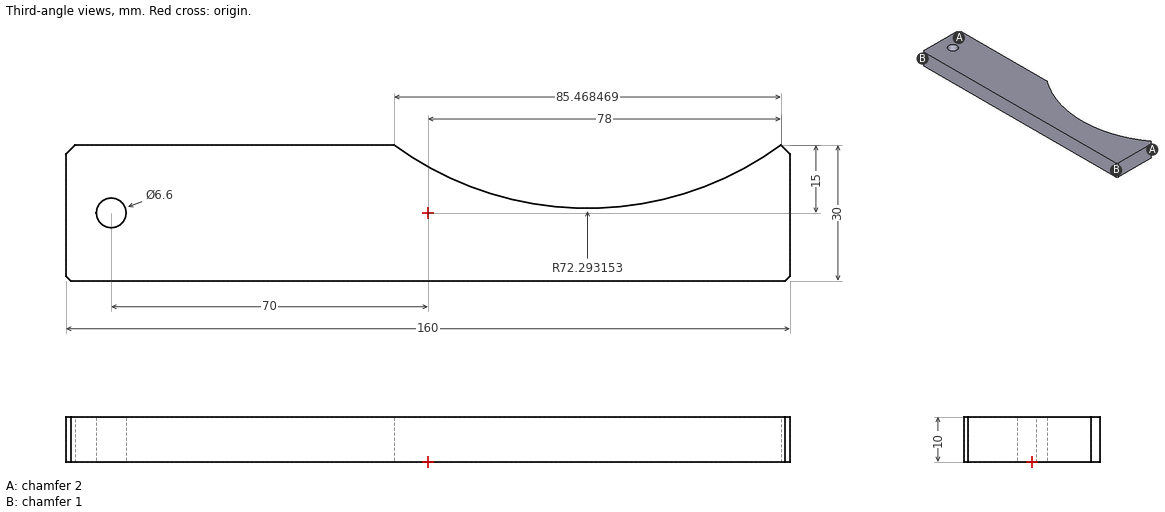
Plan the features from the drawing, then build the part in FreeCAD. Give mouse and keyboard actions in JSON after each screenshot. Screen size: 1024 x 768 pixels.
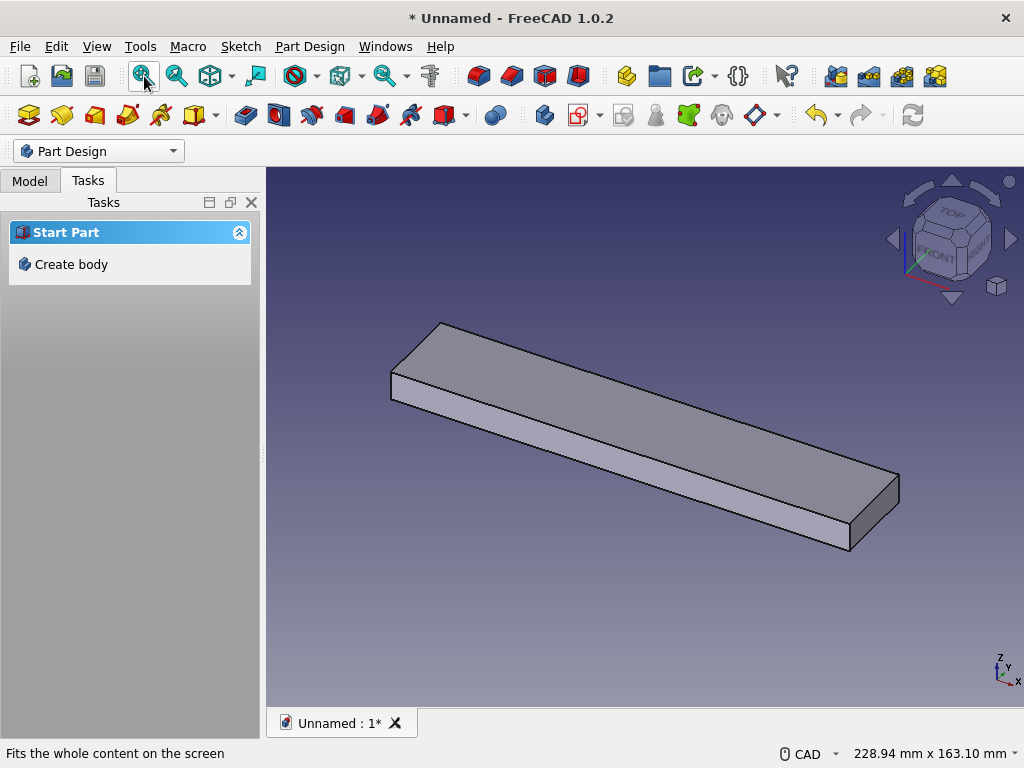
{"action": "key", "text": "0"}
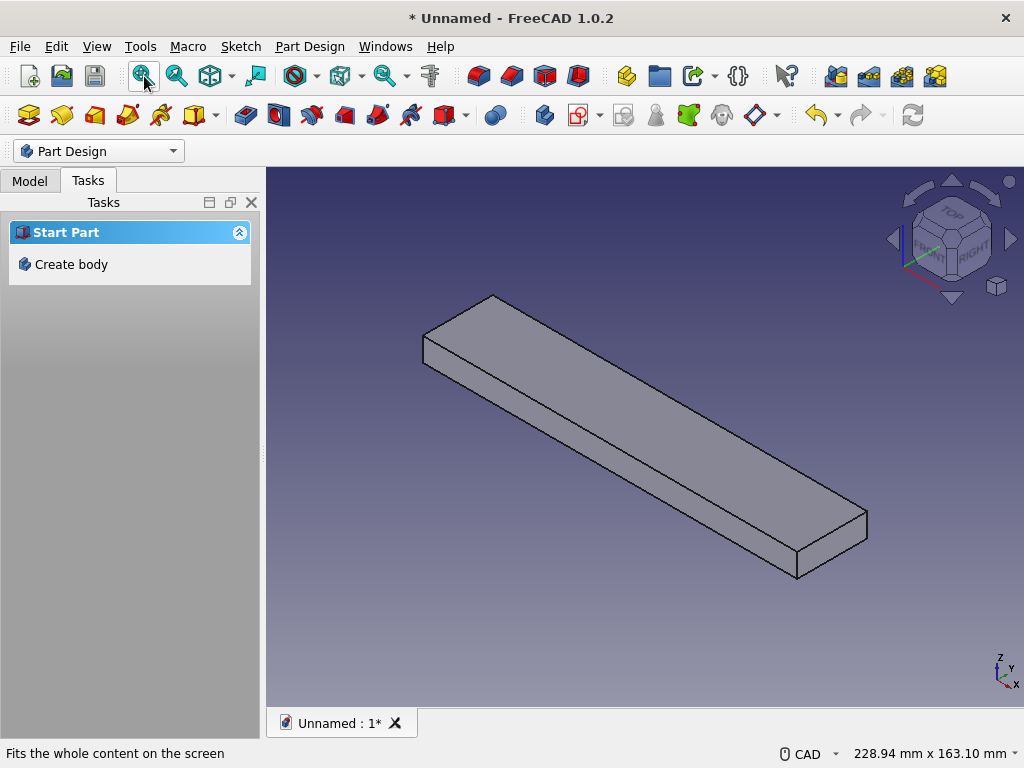
{"action": "key", "text": "2"}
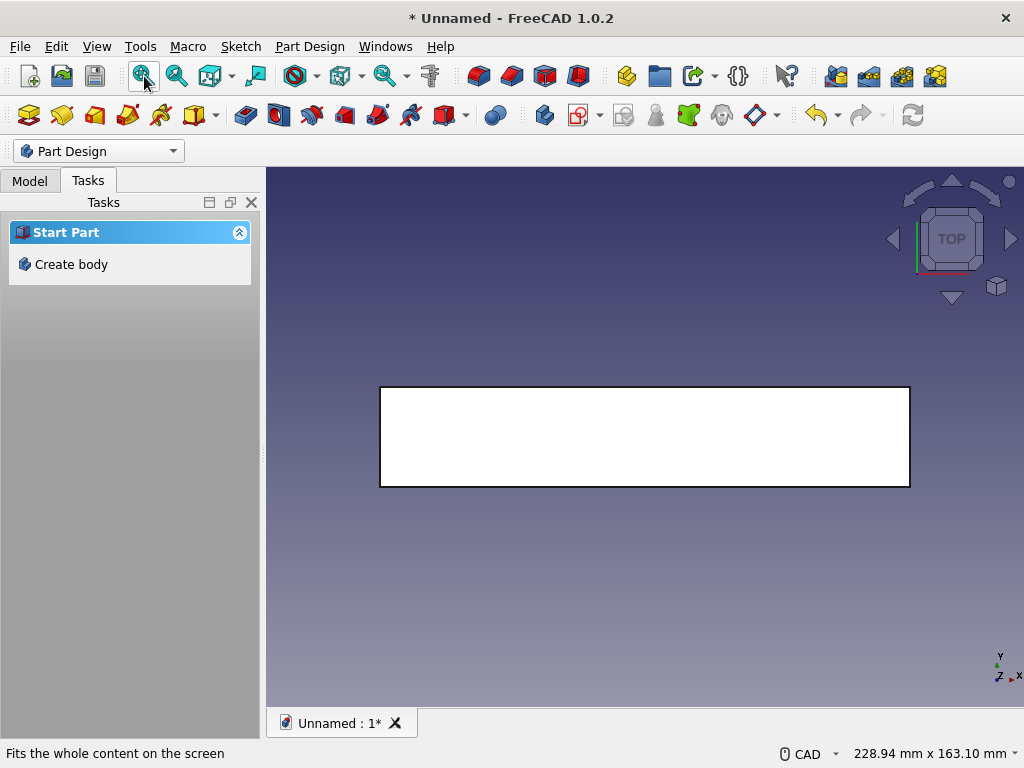
{"action": "key", "text": "1"}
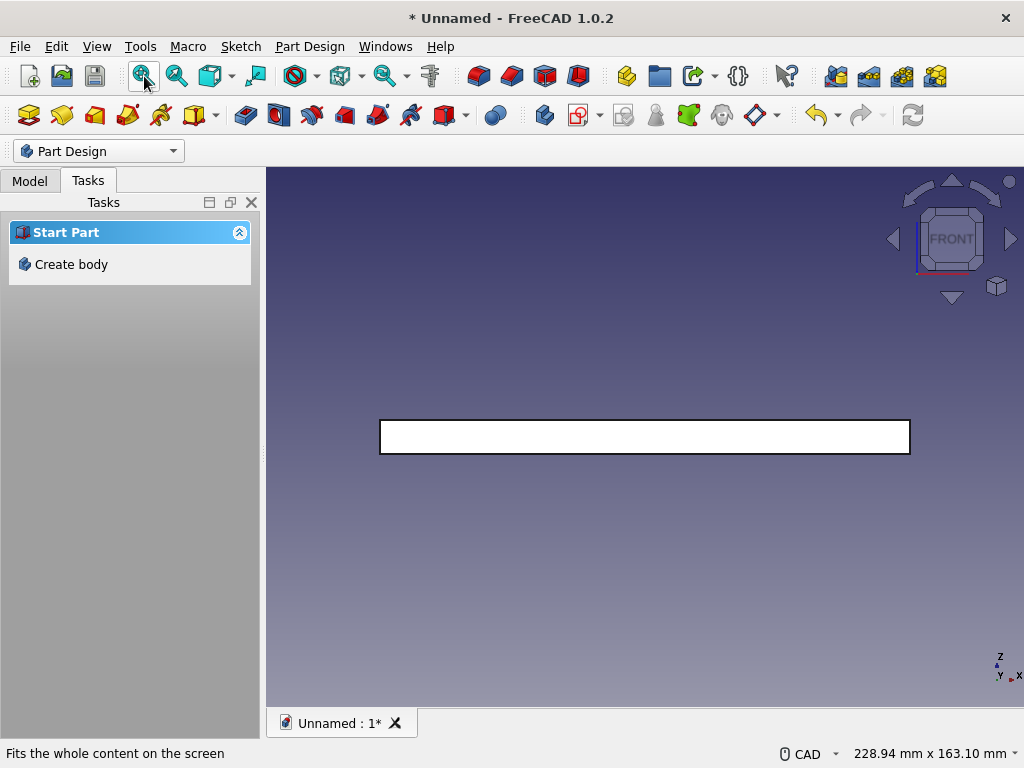
{"action": "key", "text": "3"}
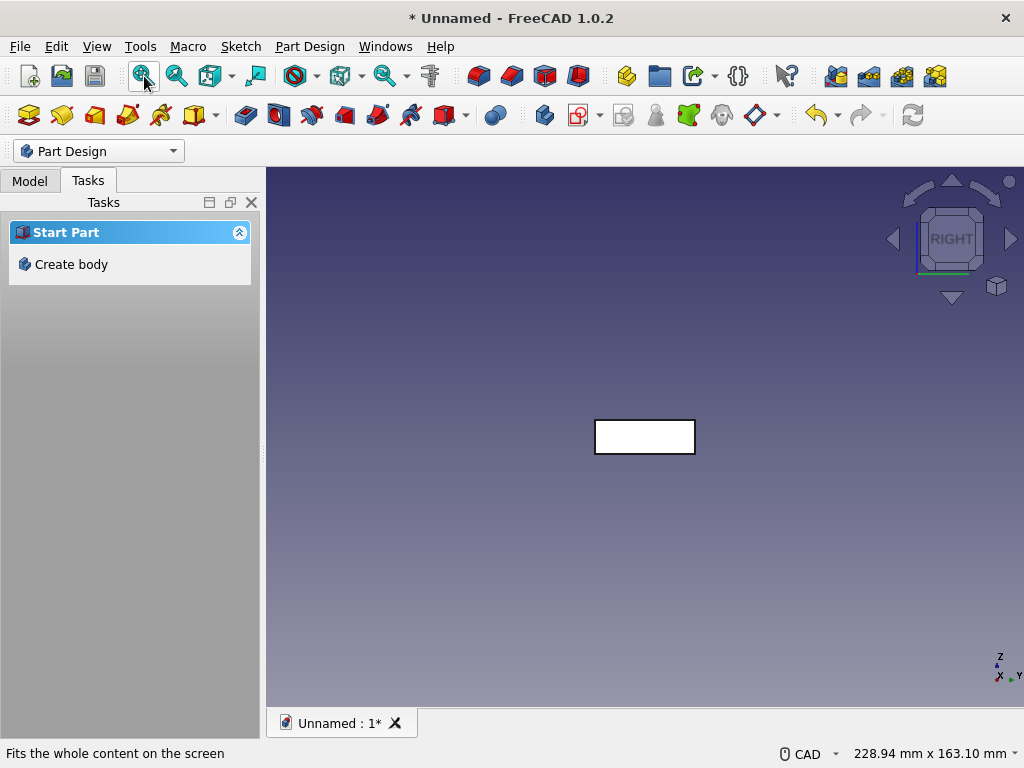
{"action": "left_click", "coordinate": [144, 76]}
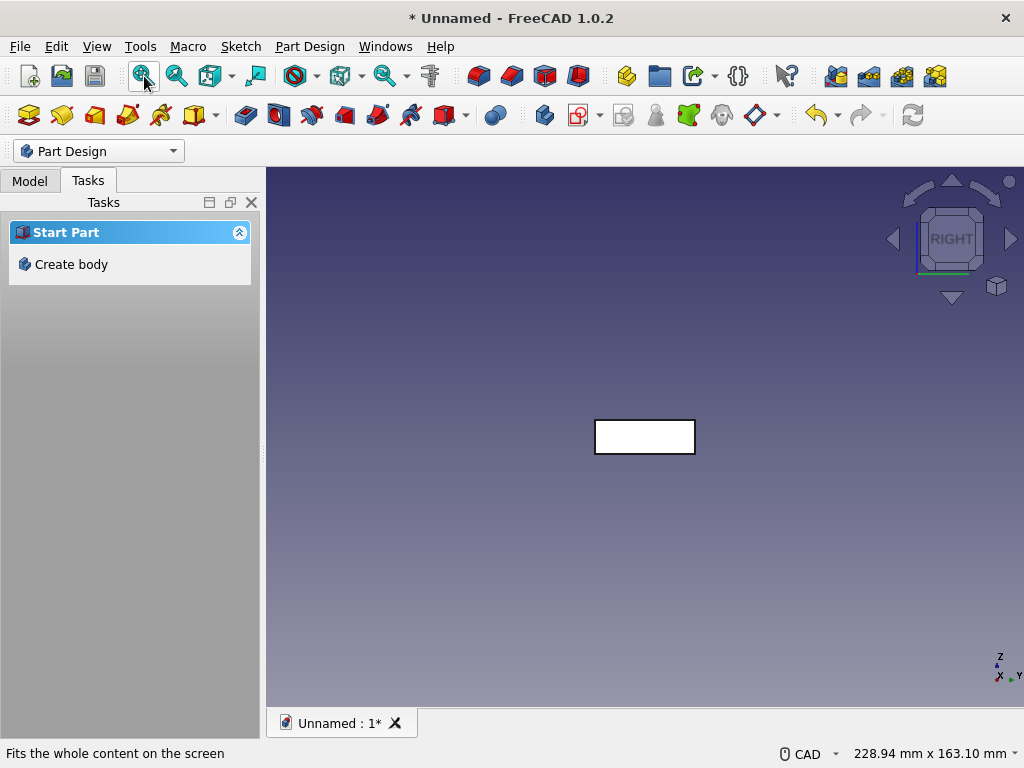
{"action": "left_click", "coordinate": [695, 436]}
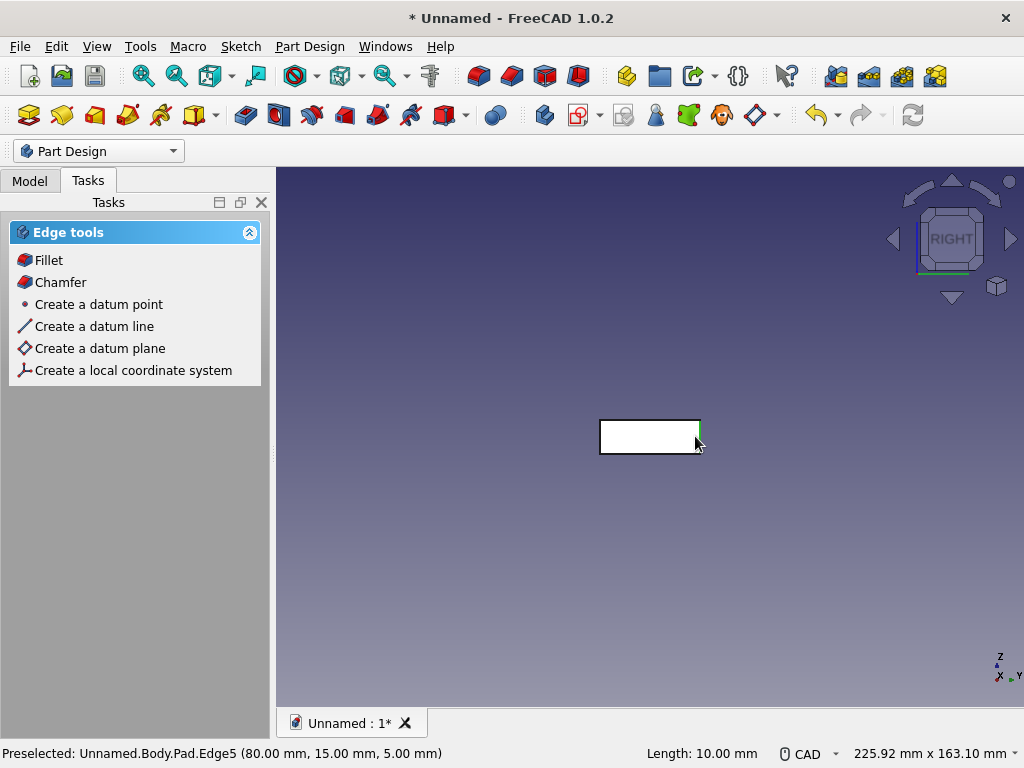
{"action": "key", "text": "5"}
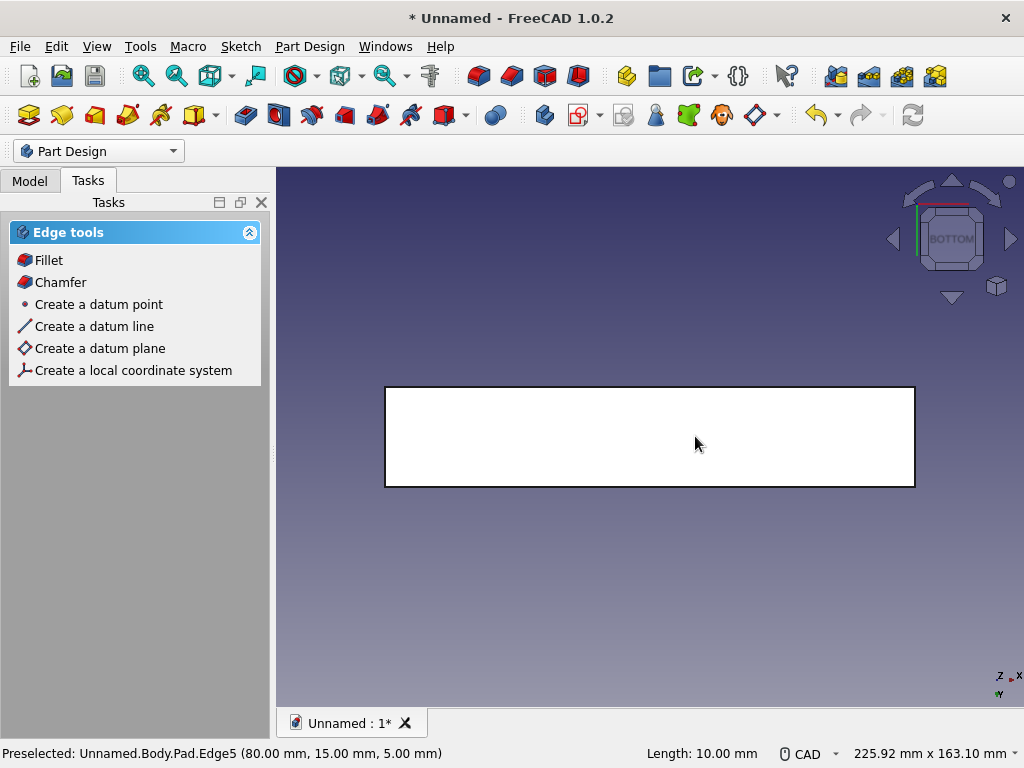
{"action": "key", "text": "4"}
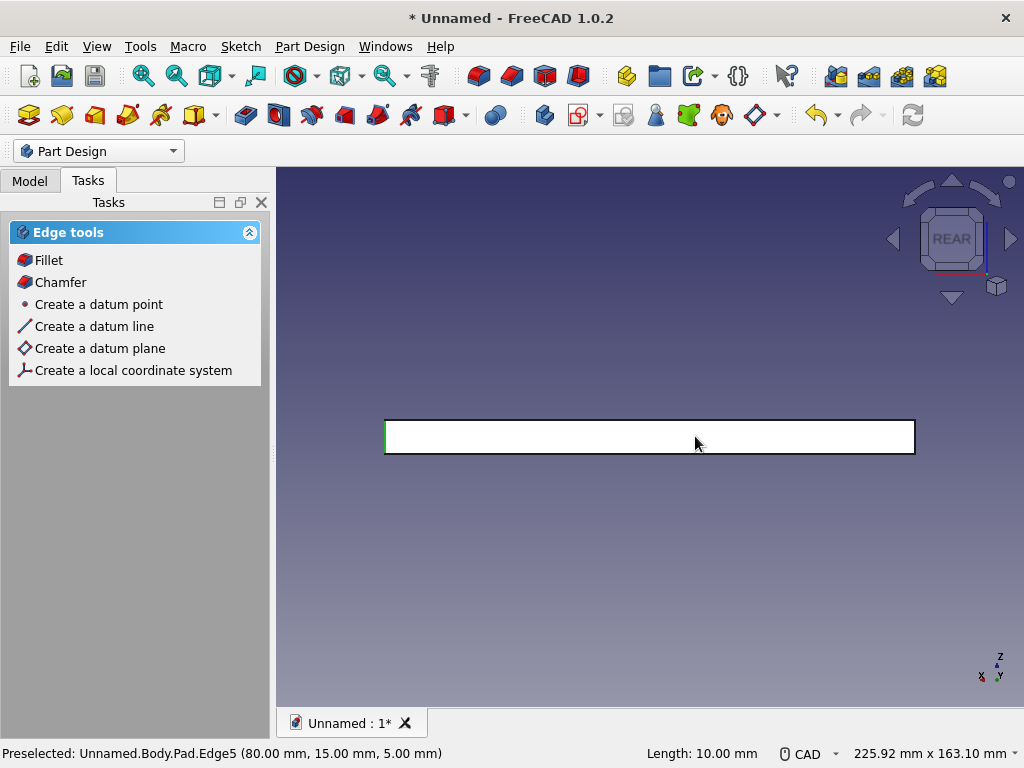
{"action": "left_click", "coordinate": [915, 436], "text": "ctrl"}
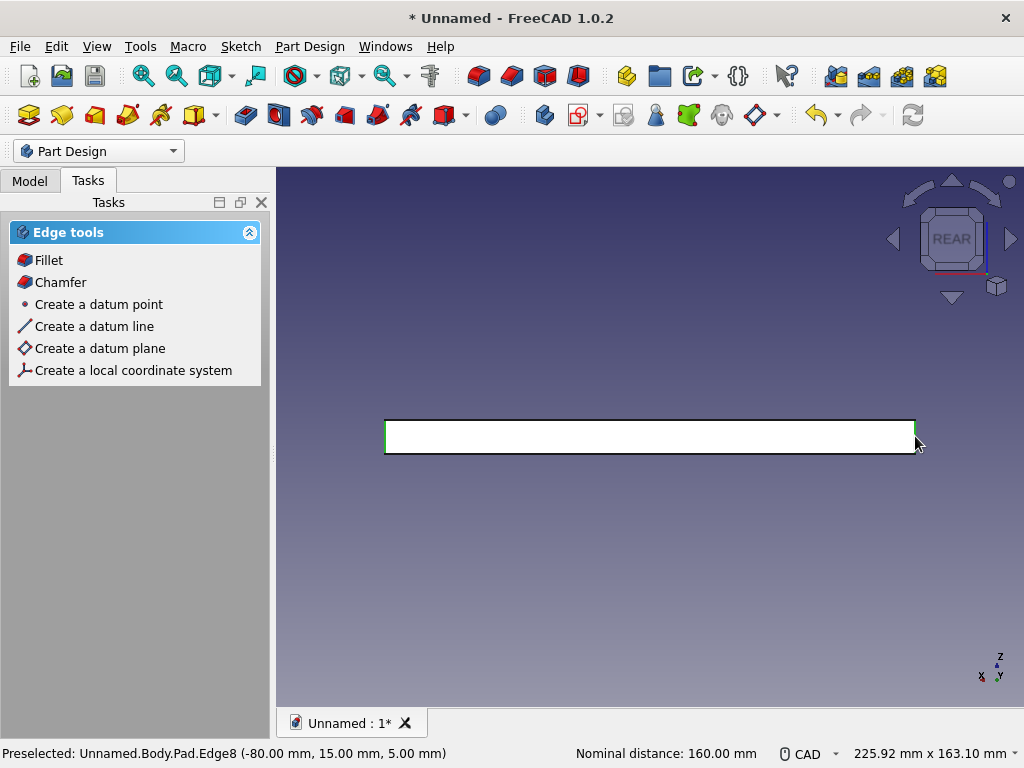
{"action": "left_click", "coordinate": [512, 76]}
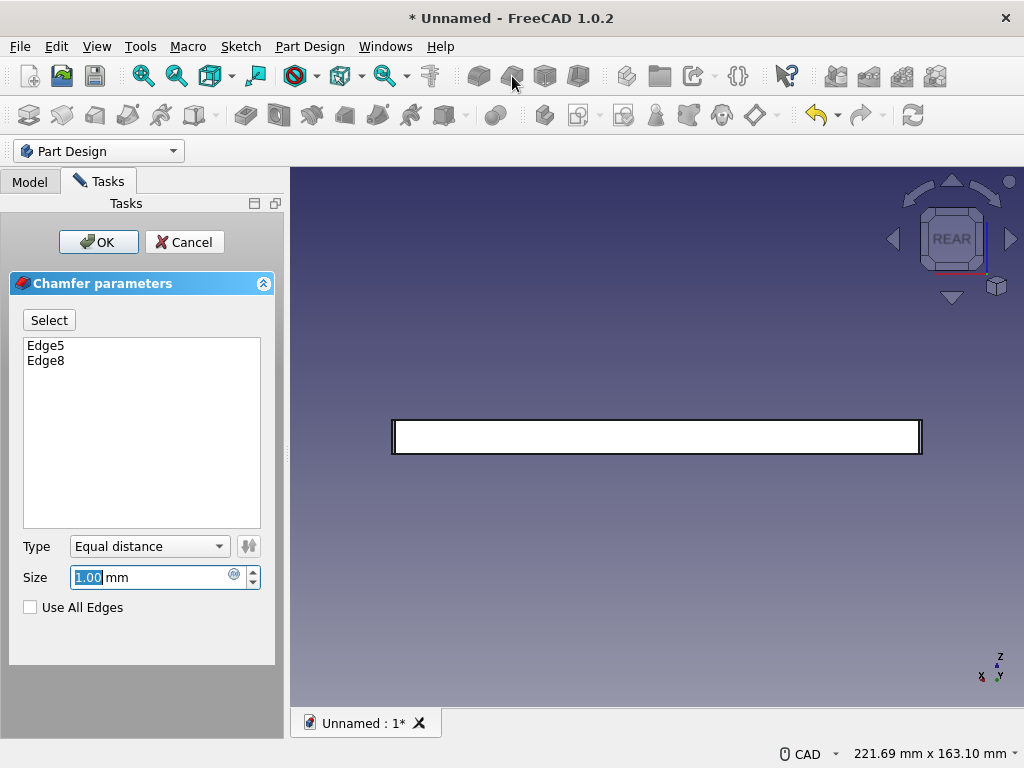
{"action": "type", "text": "2"}
{"action": "key", "text": "Tab"}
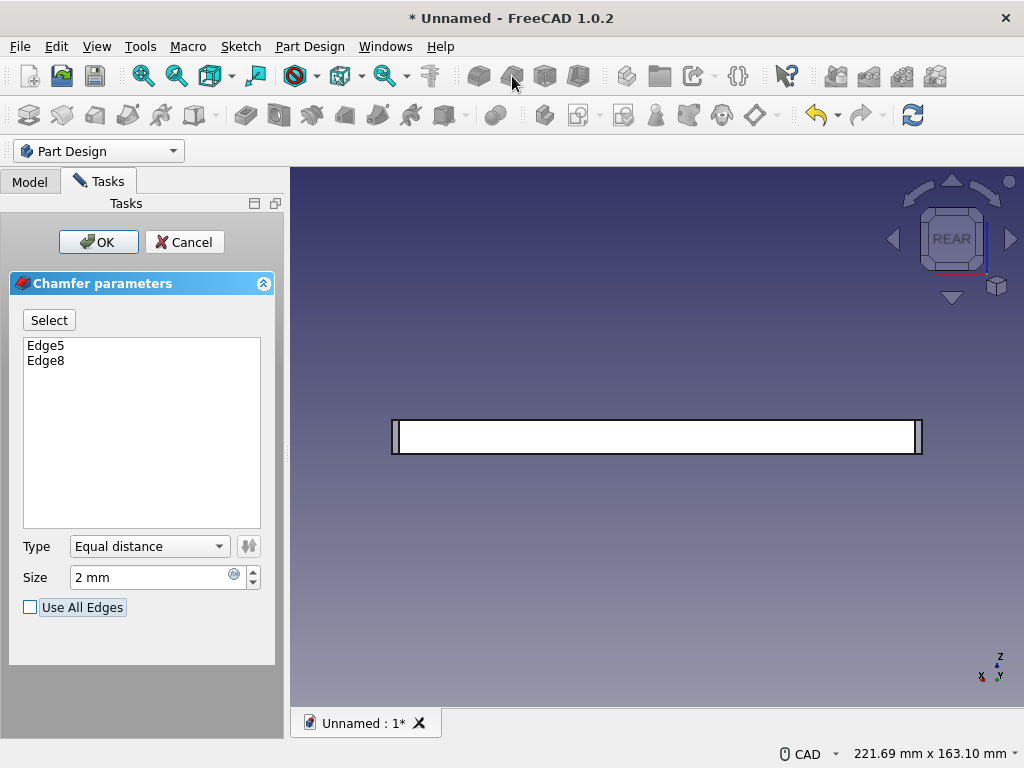
{"action": "left_click", "coordinate": [99, 242]}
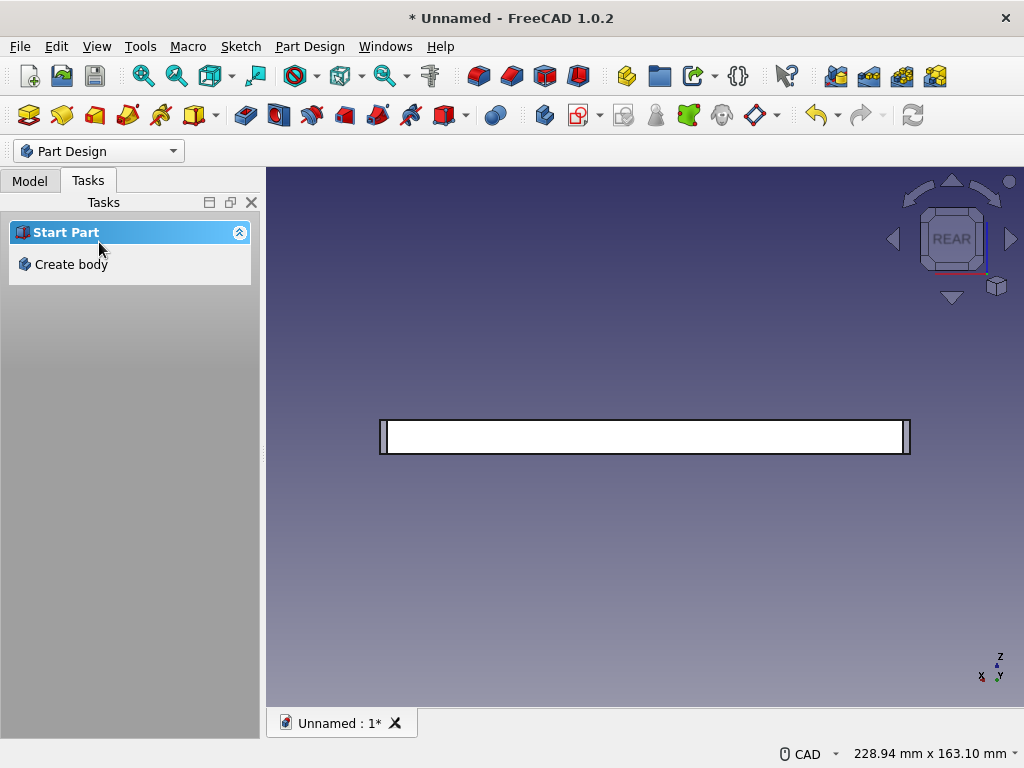
{"action": "key", "text": "0"}